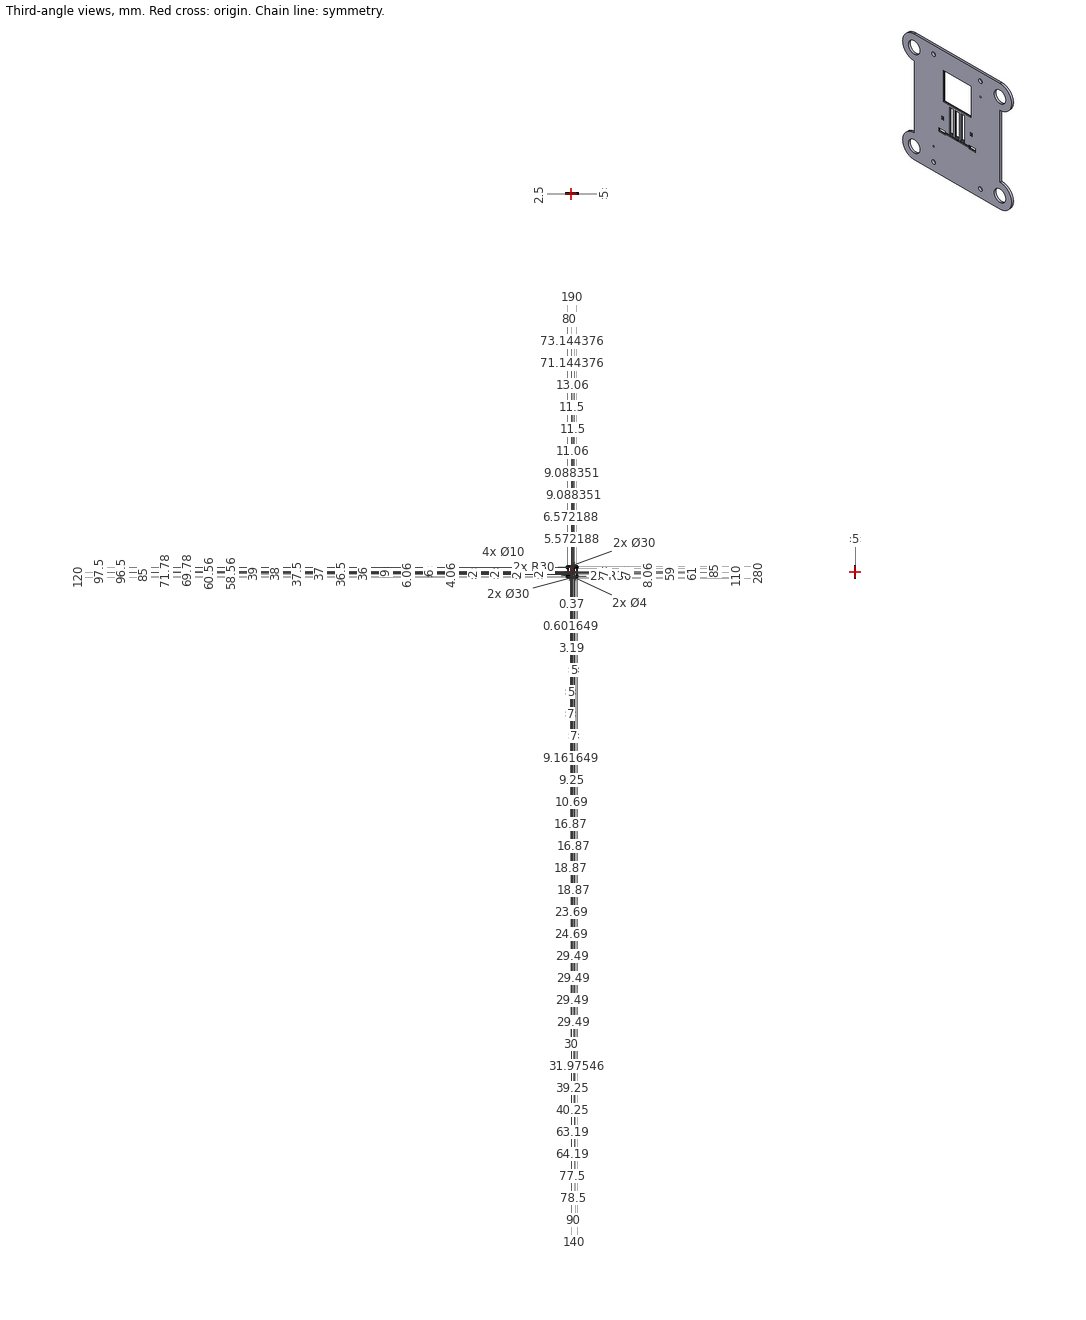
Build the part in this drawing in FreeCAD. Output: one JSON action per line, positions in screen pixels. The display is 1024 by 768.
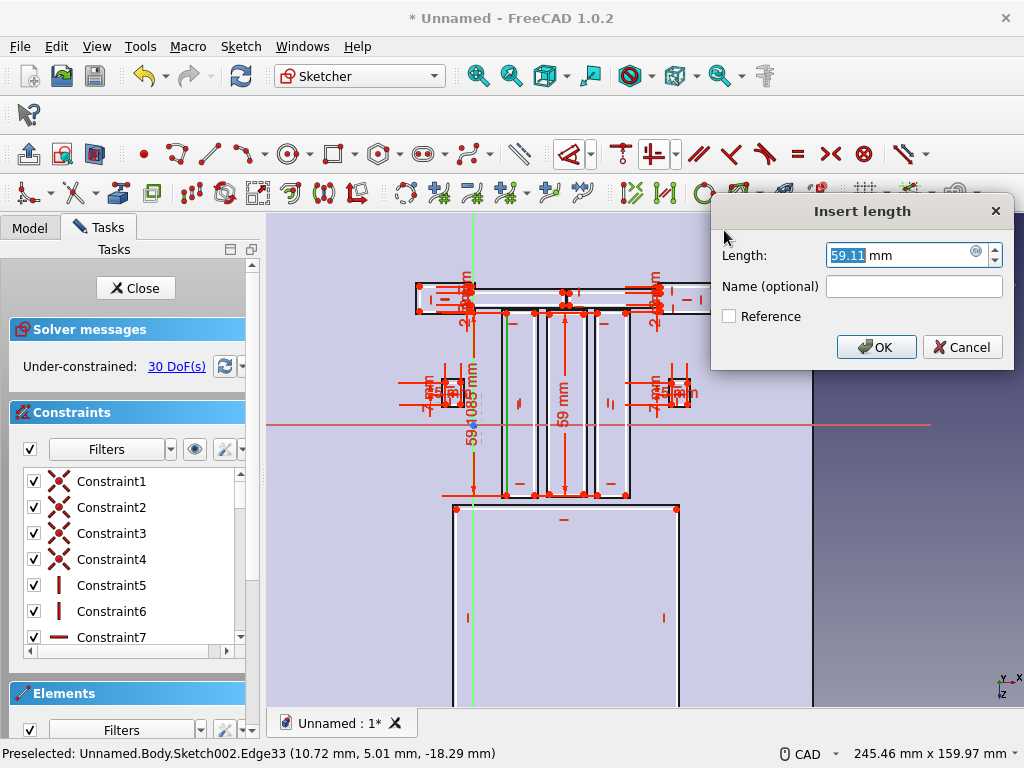
{"action": "type", "text": "59"}
{"action": "key", "text": "Return"}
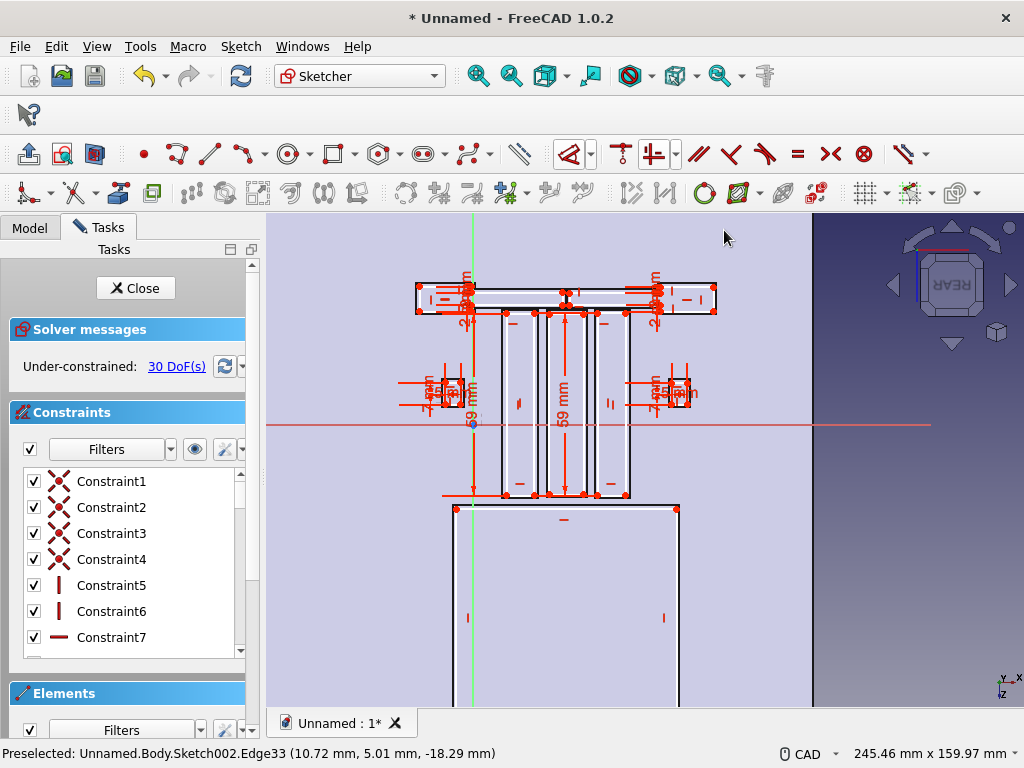
{"action": "scroll", "coordinate": [672, 405], "scroll_direction": "up", "scroll_amount": 4}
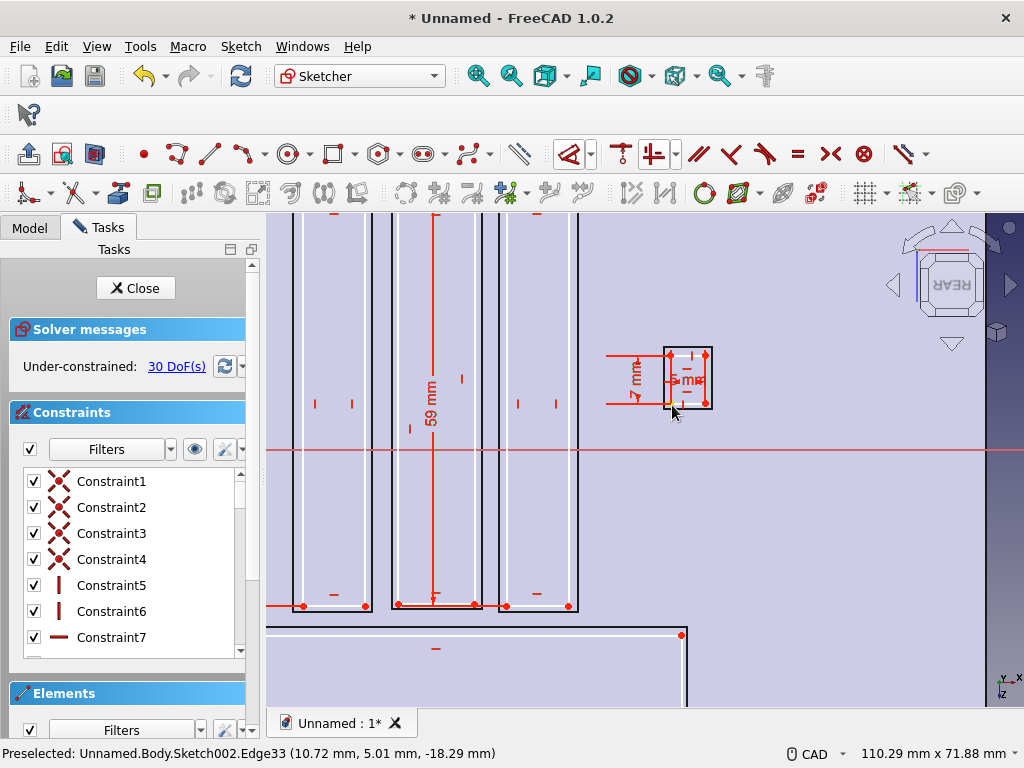
{"action": "left_click", "coordinate": [671, 404]}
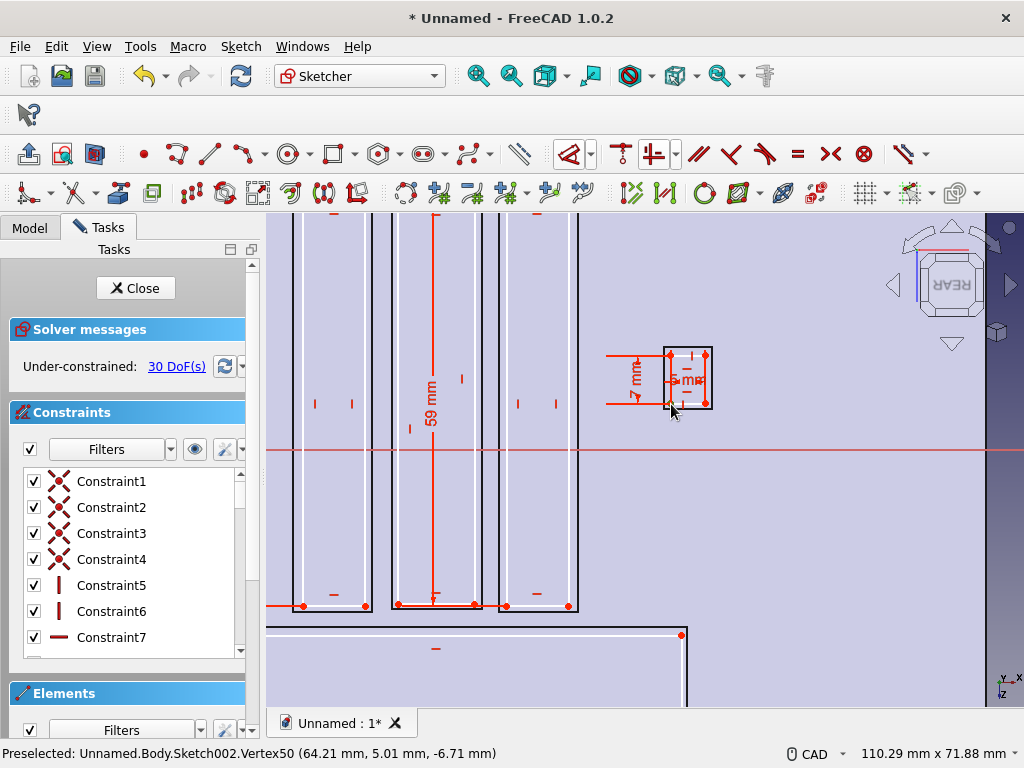
{"action": "key", "text": "i"}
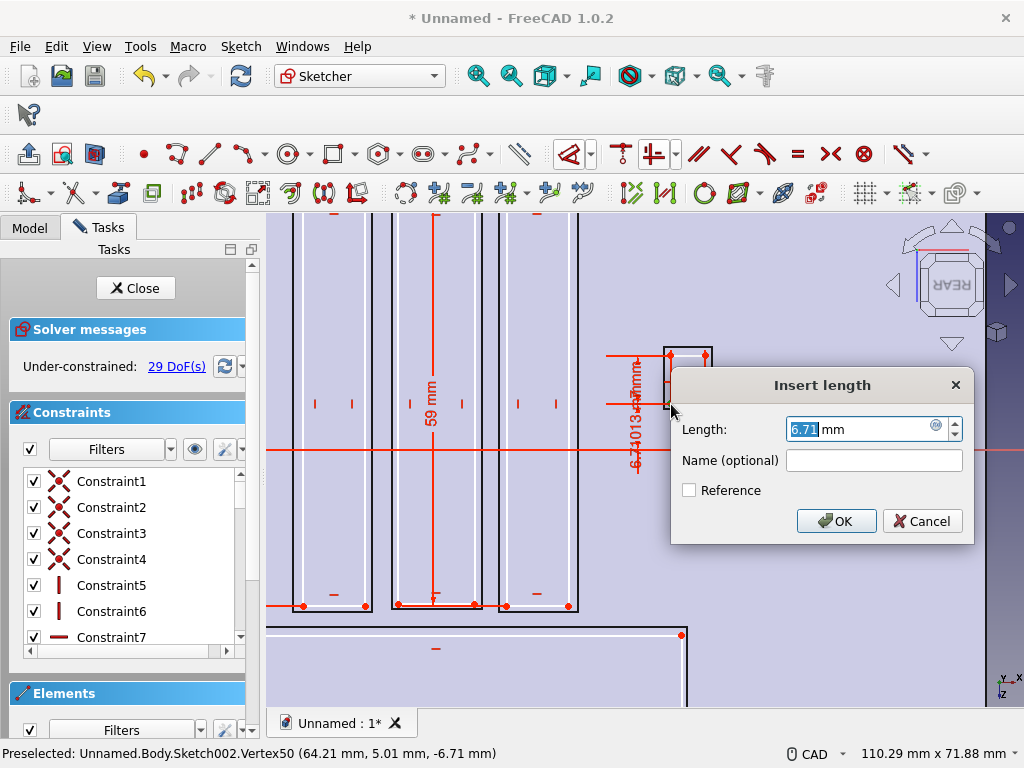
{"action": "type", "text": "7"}
{"action": "key", "text": "Return"}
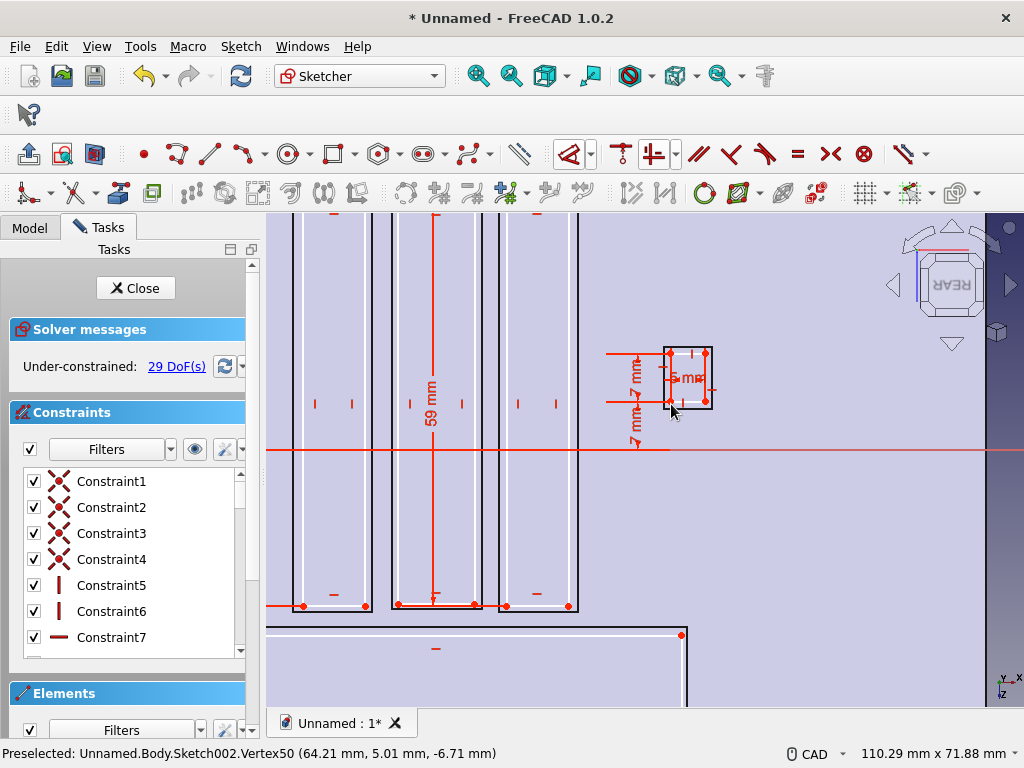
{"action": "scroll", "coordinate": [637, 388], "scroll_direction": "down", "scroll_amount": 6}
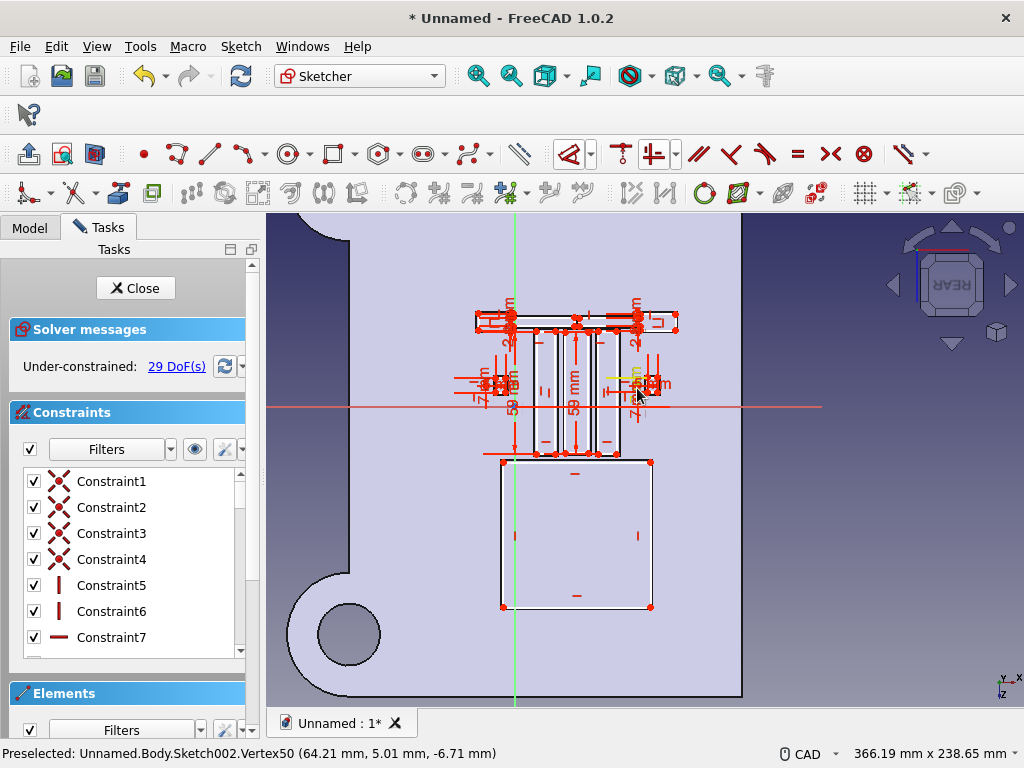
{"action": "scroll", "coordinate": [496, 393], "scroll_direction": "up", "scroll_amount": 6}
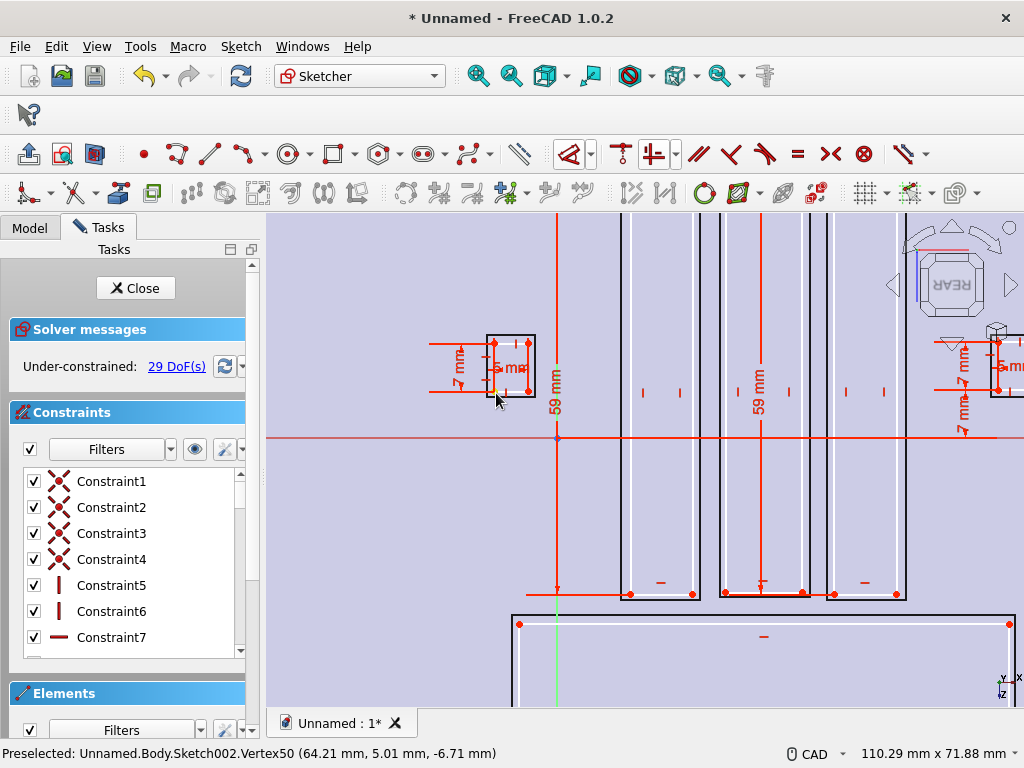
{"action": "left_click", "coordinate": [494, 392]}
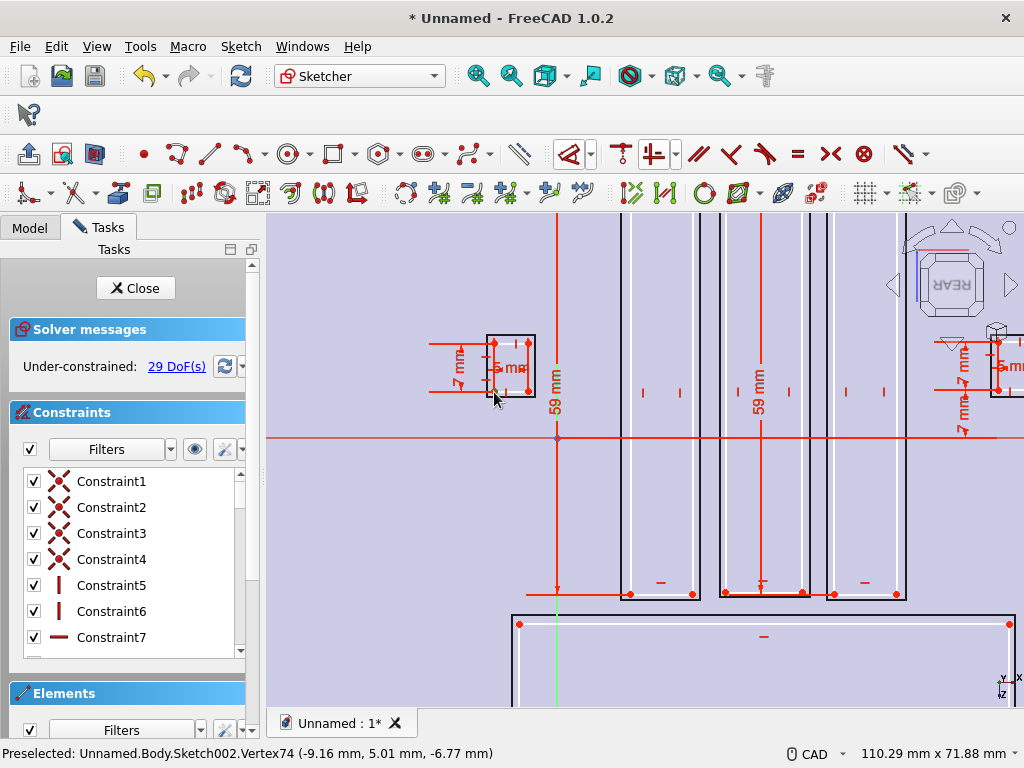
{"action": "left_click", "coordinate": [590, 154]}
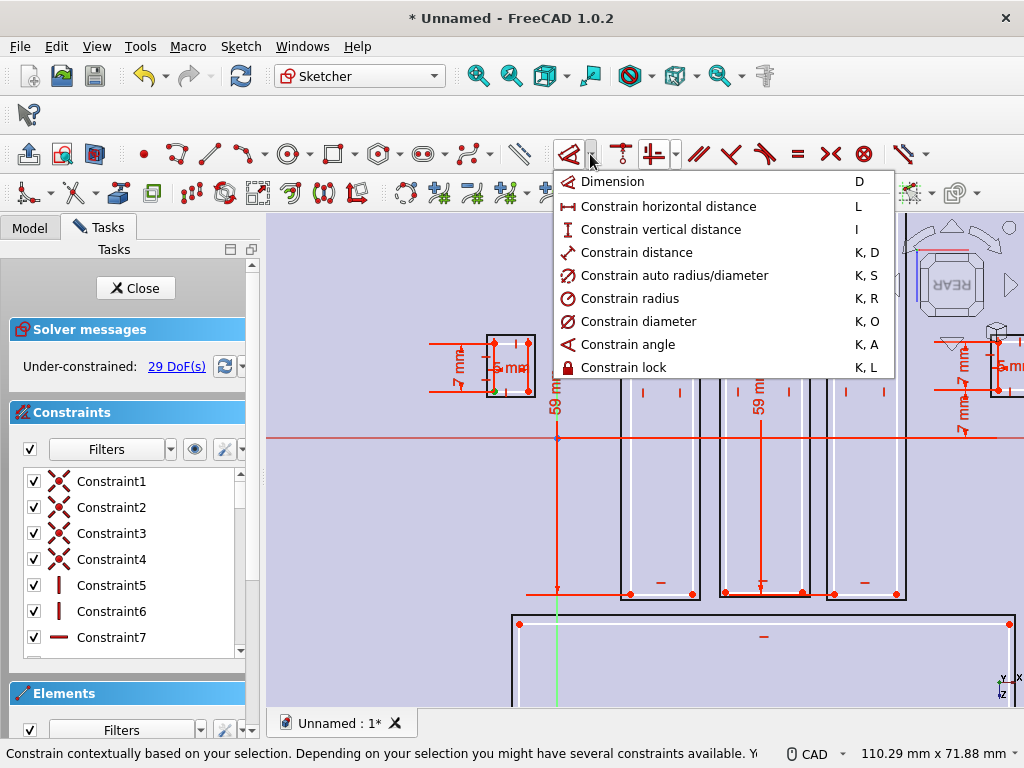
{"action": "left_click", "coordinate": [724, 230]}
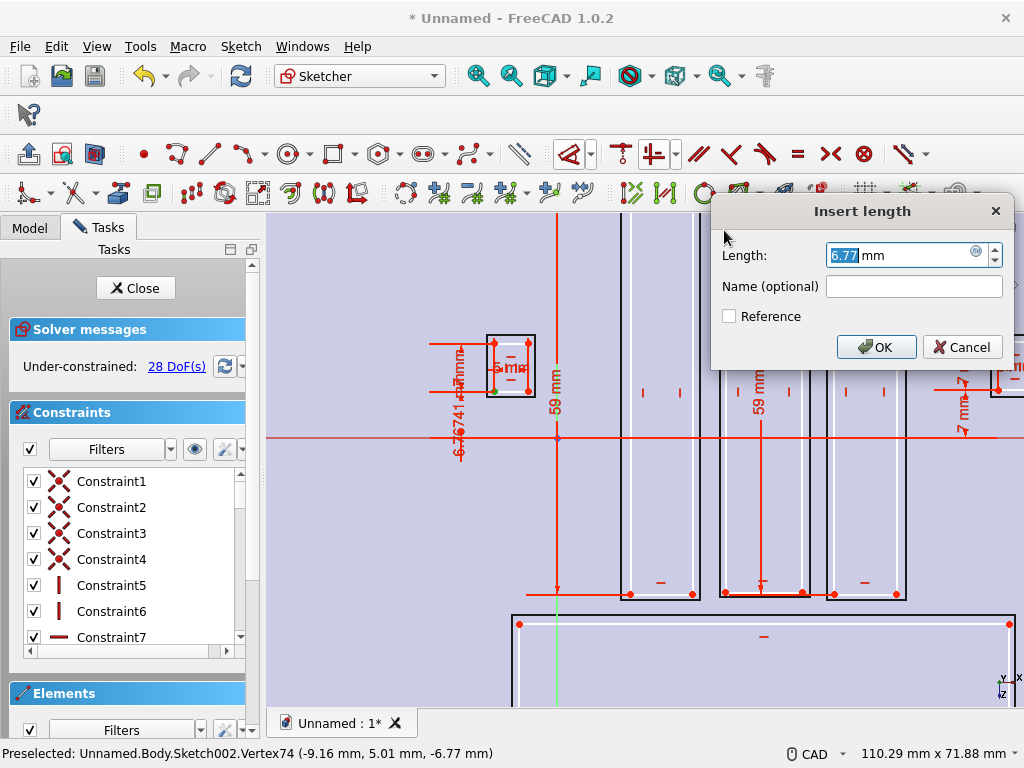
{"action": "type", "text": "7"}
{"action": "key", "text": "Return"}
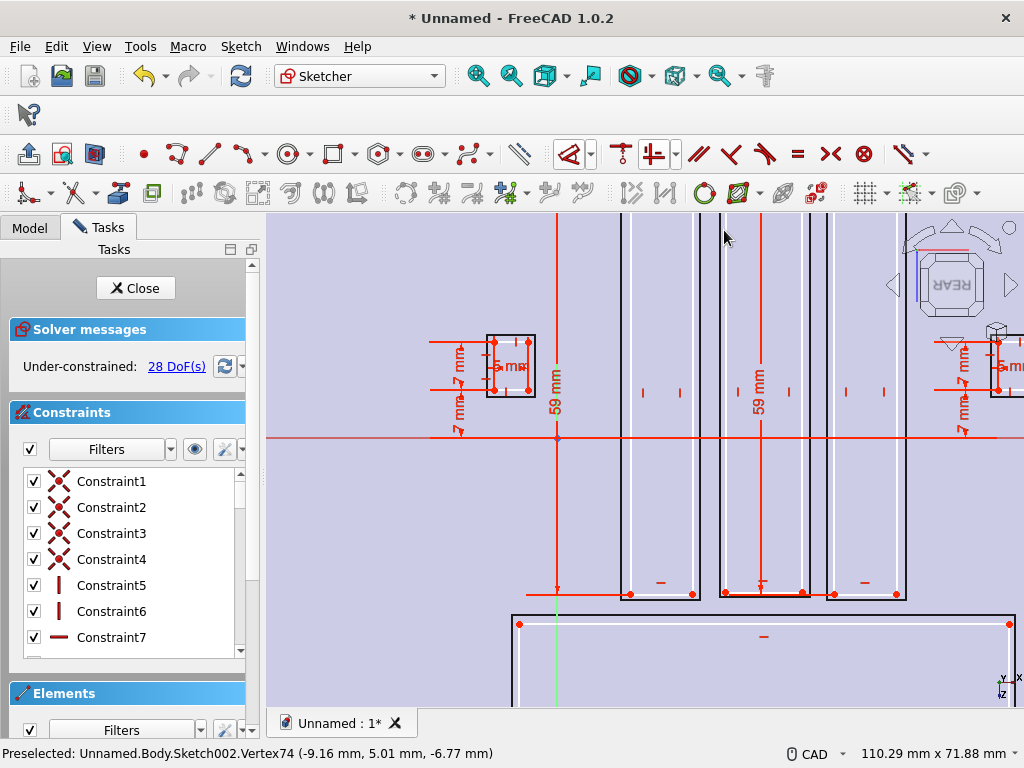
{"action": "scroll", "coordinate": [496, 393], "scroll_direction": "down", "scroll_amount": 6}